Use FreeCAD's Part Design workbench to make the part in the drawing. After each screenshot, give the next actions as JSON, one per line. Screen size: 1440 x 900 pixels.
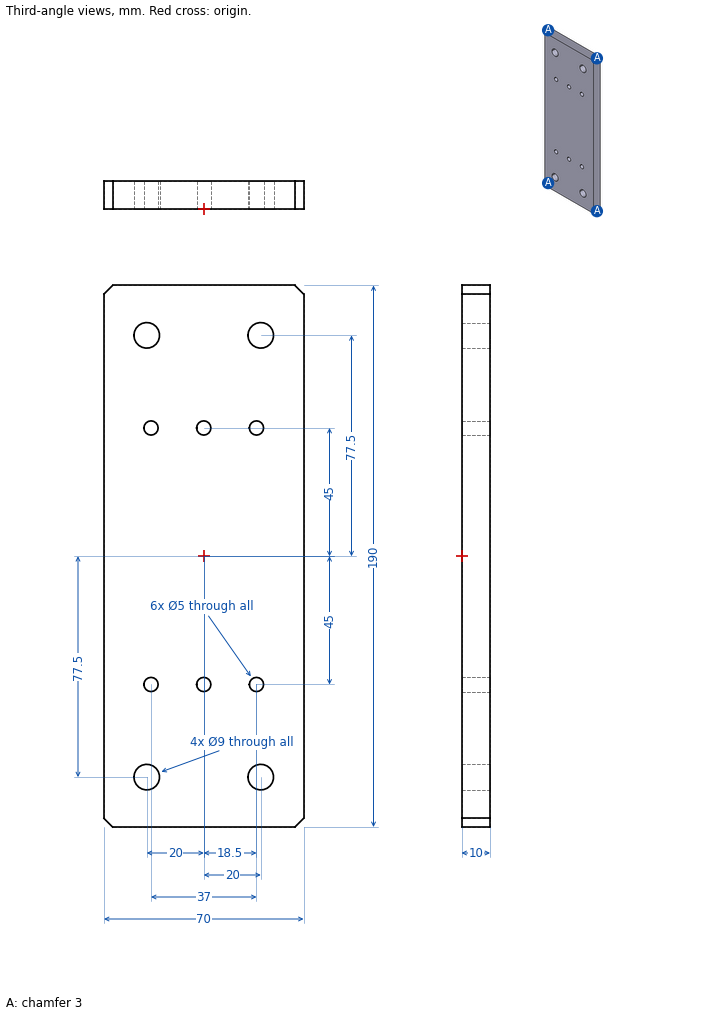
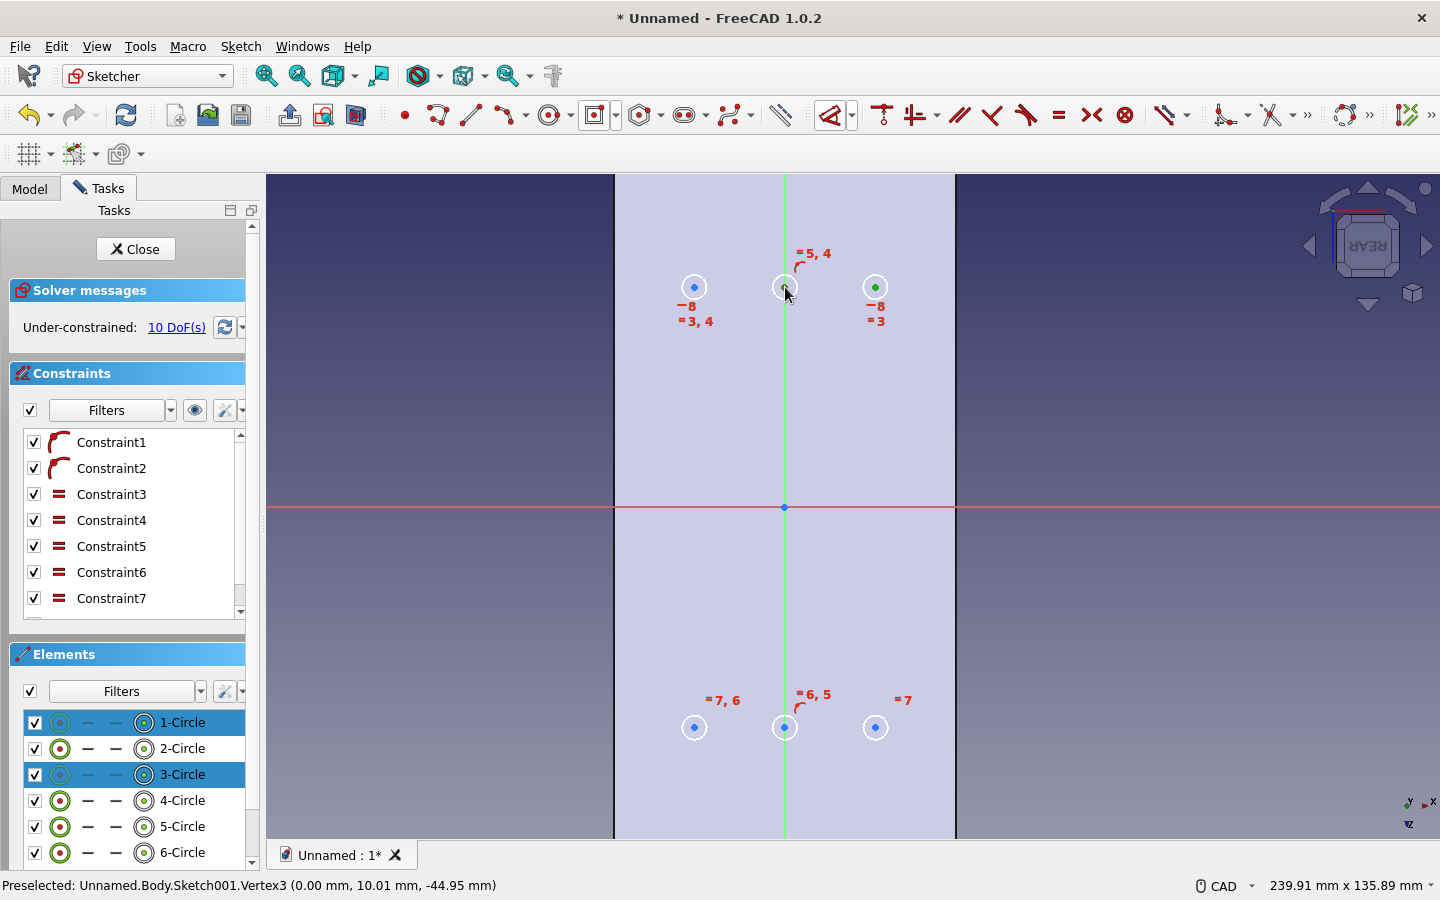
{"action": "left_click", "coordinate": [936, 116]}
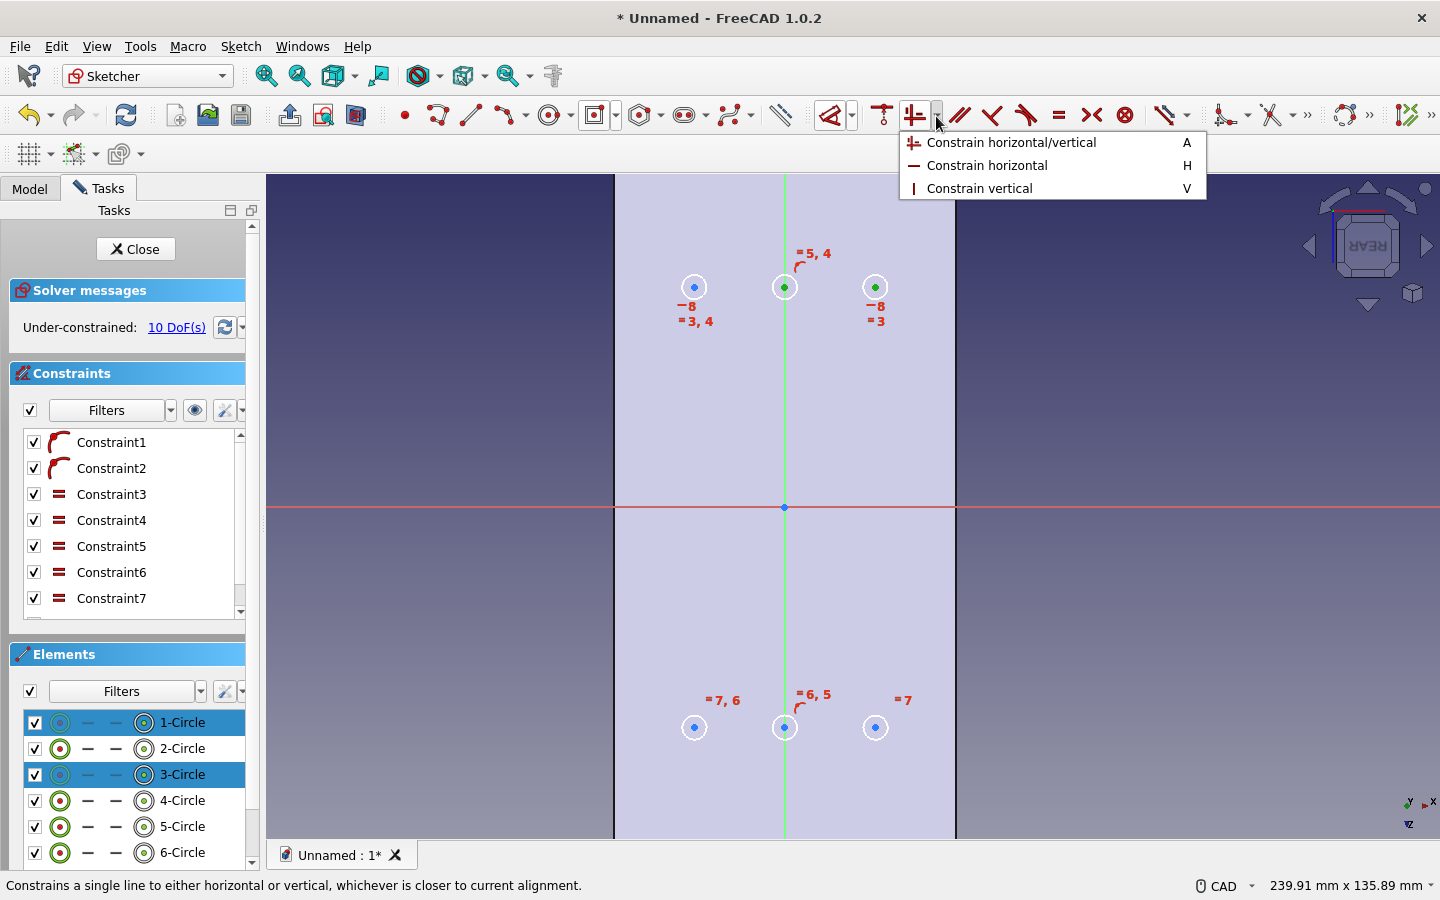
{"action": "left_click", "coordinate": [1053, 166]}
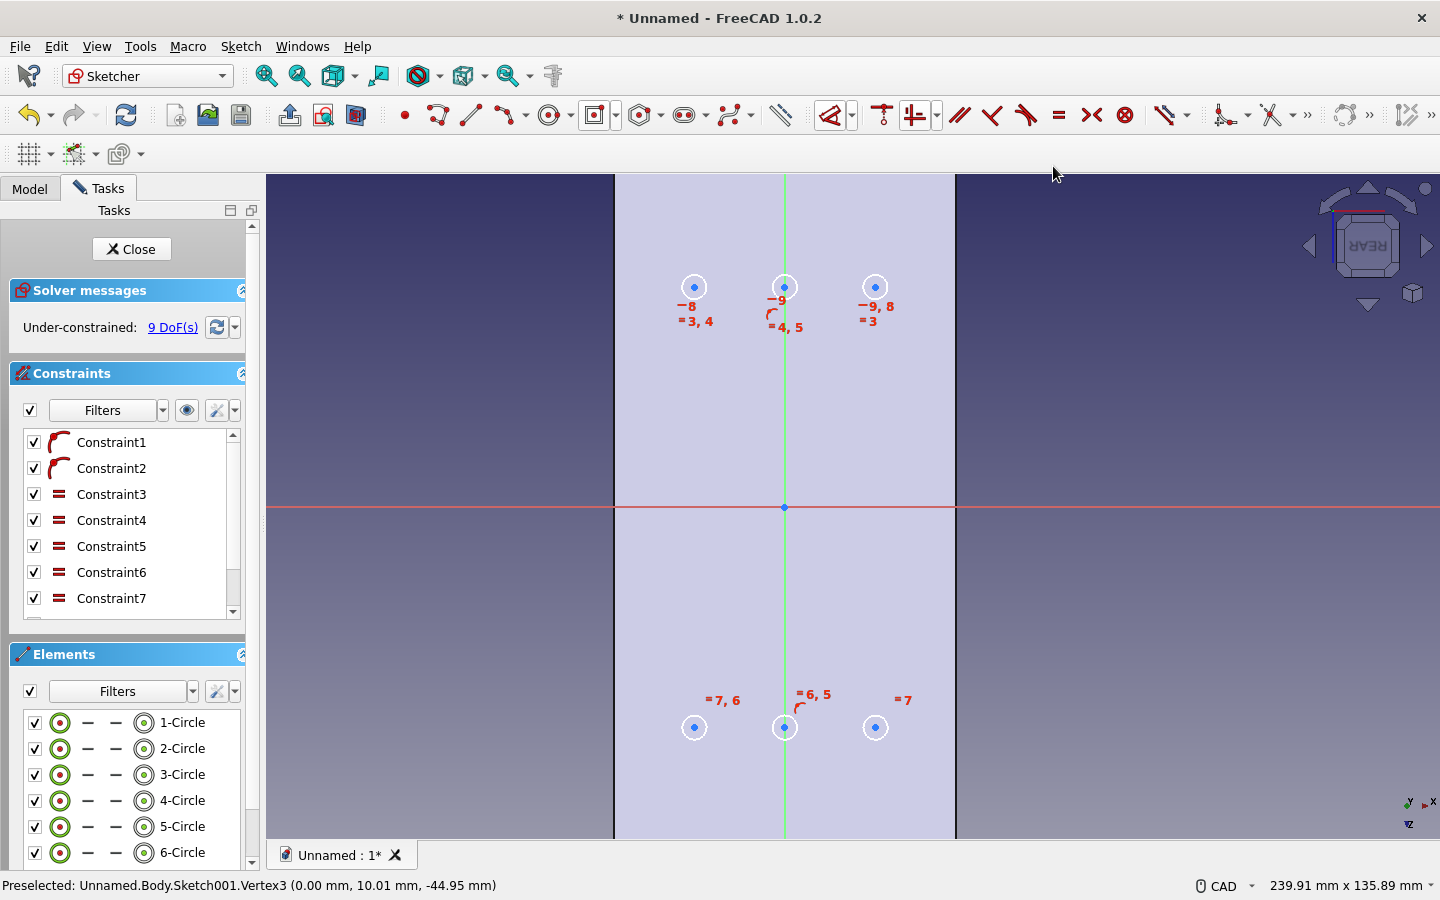
{"action": "left_click", "coordinate": [694, 287]}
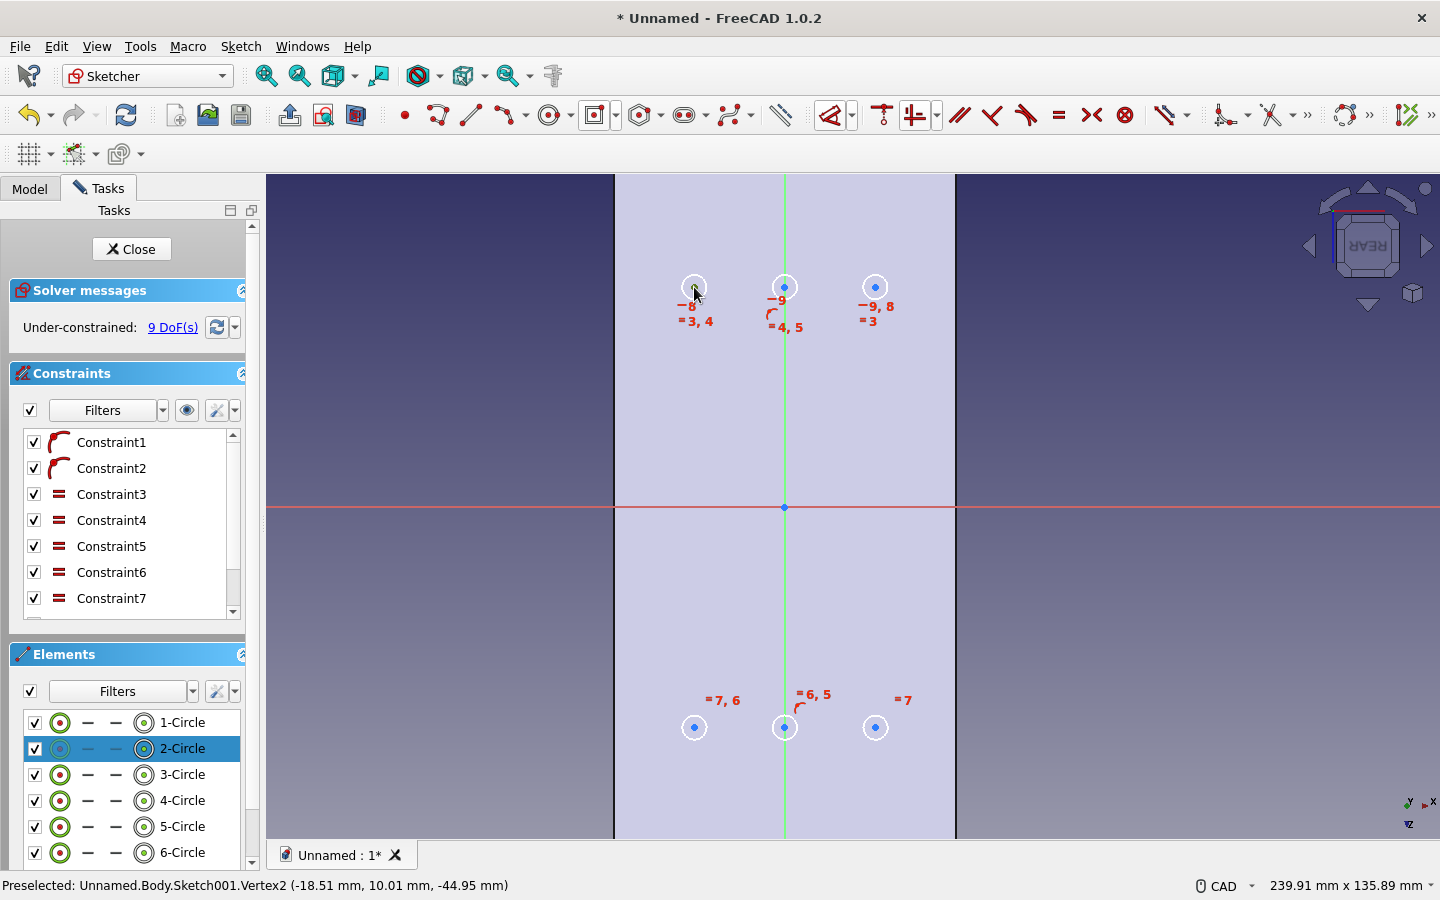
{"action": "left_click", "coordinate": [694, 728]}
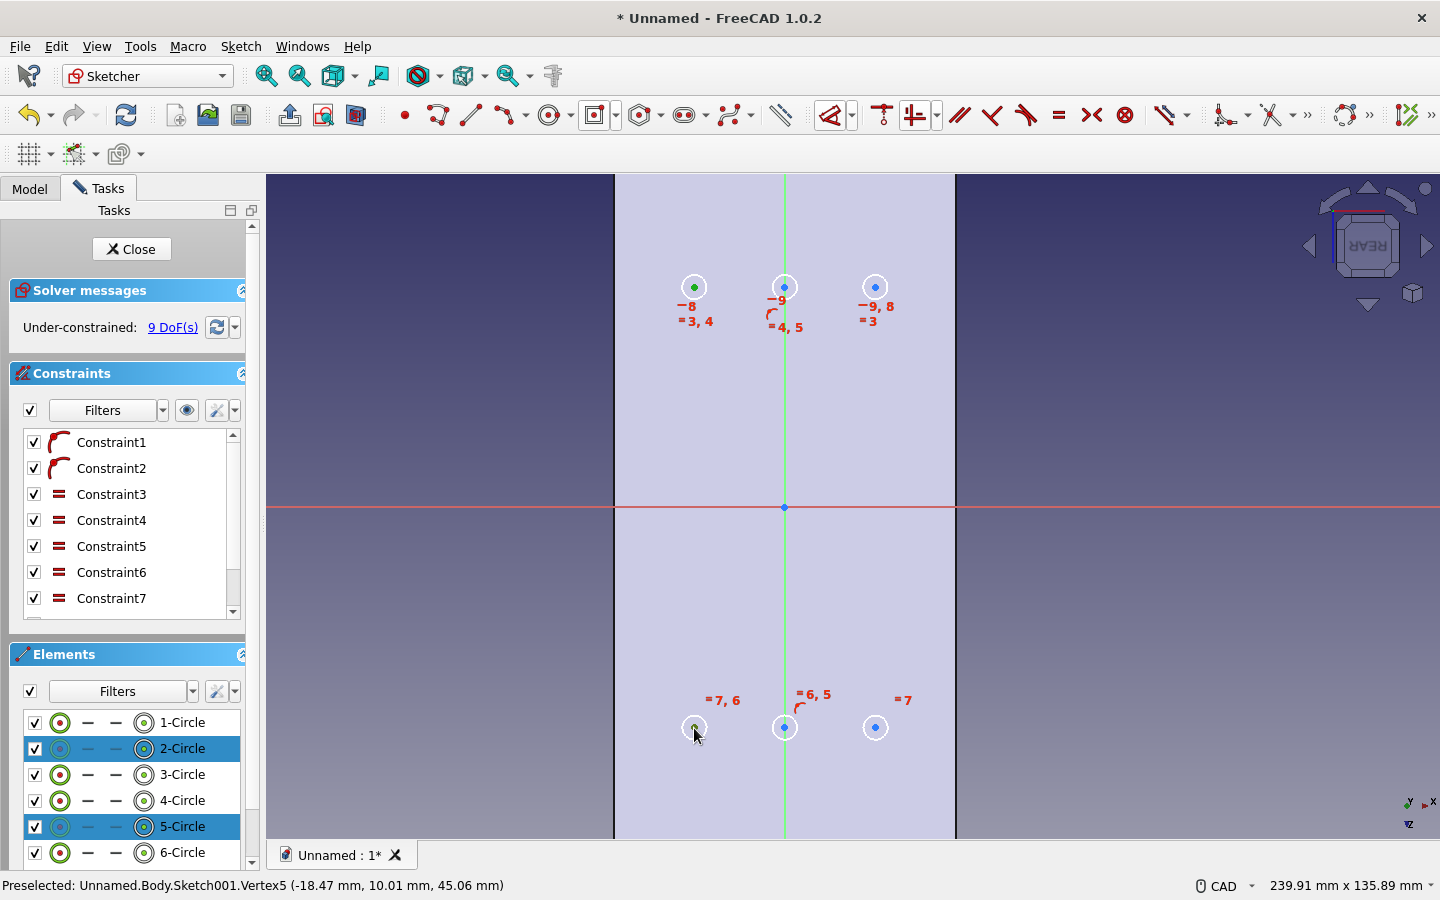
{"action": "key", "text": "v"}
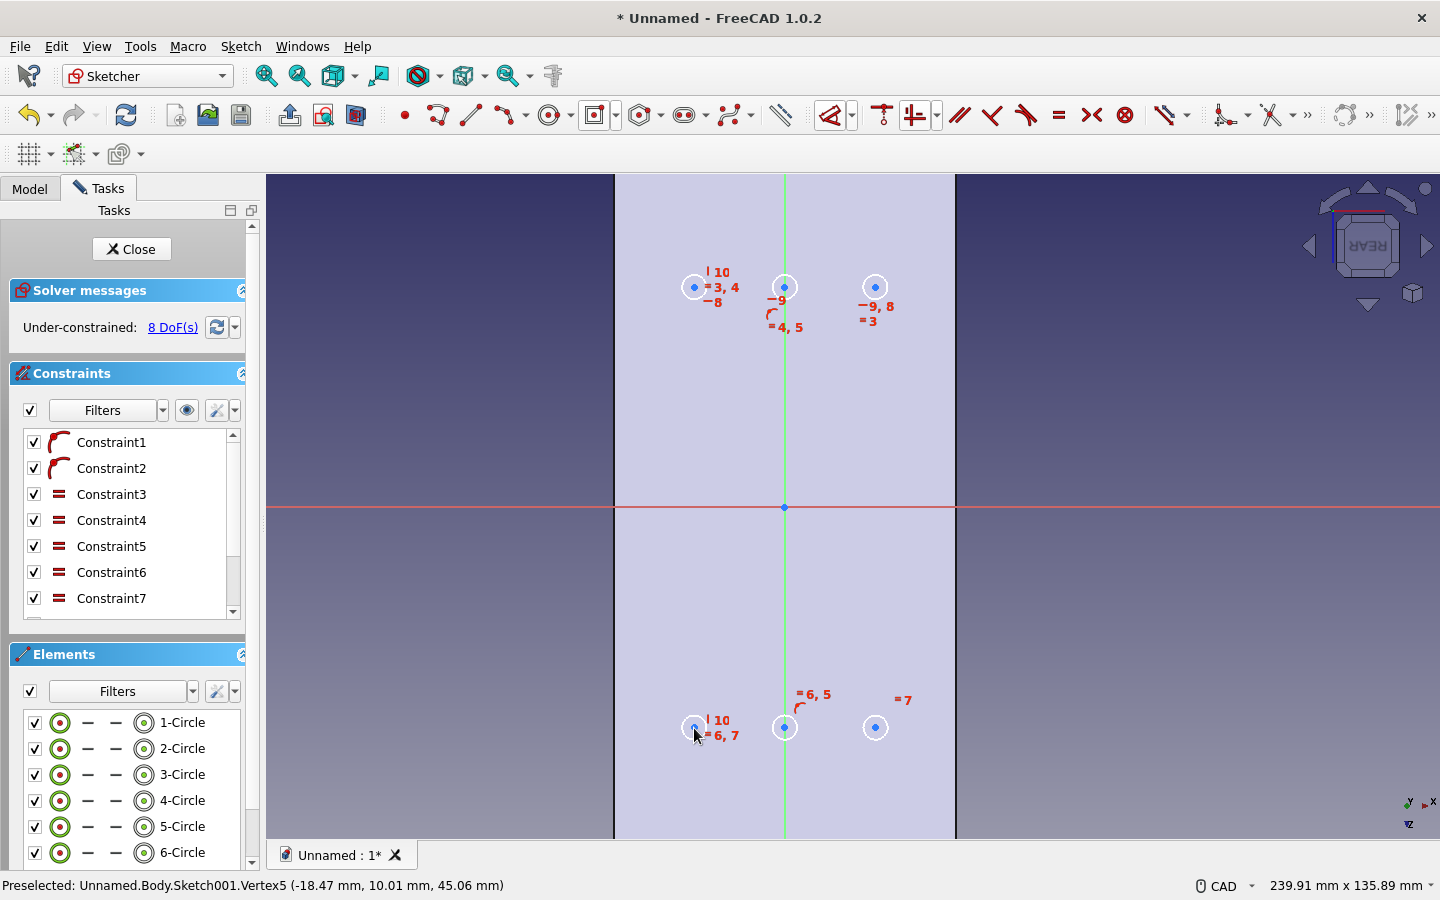
{"action": "left_click", "coordinate": [785, 728]}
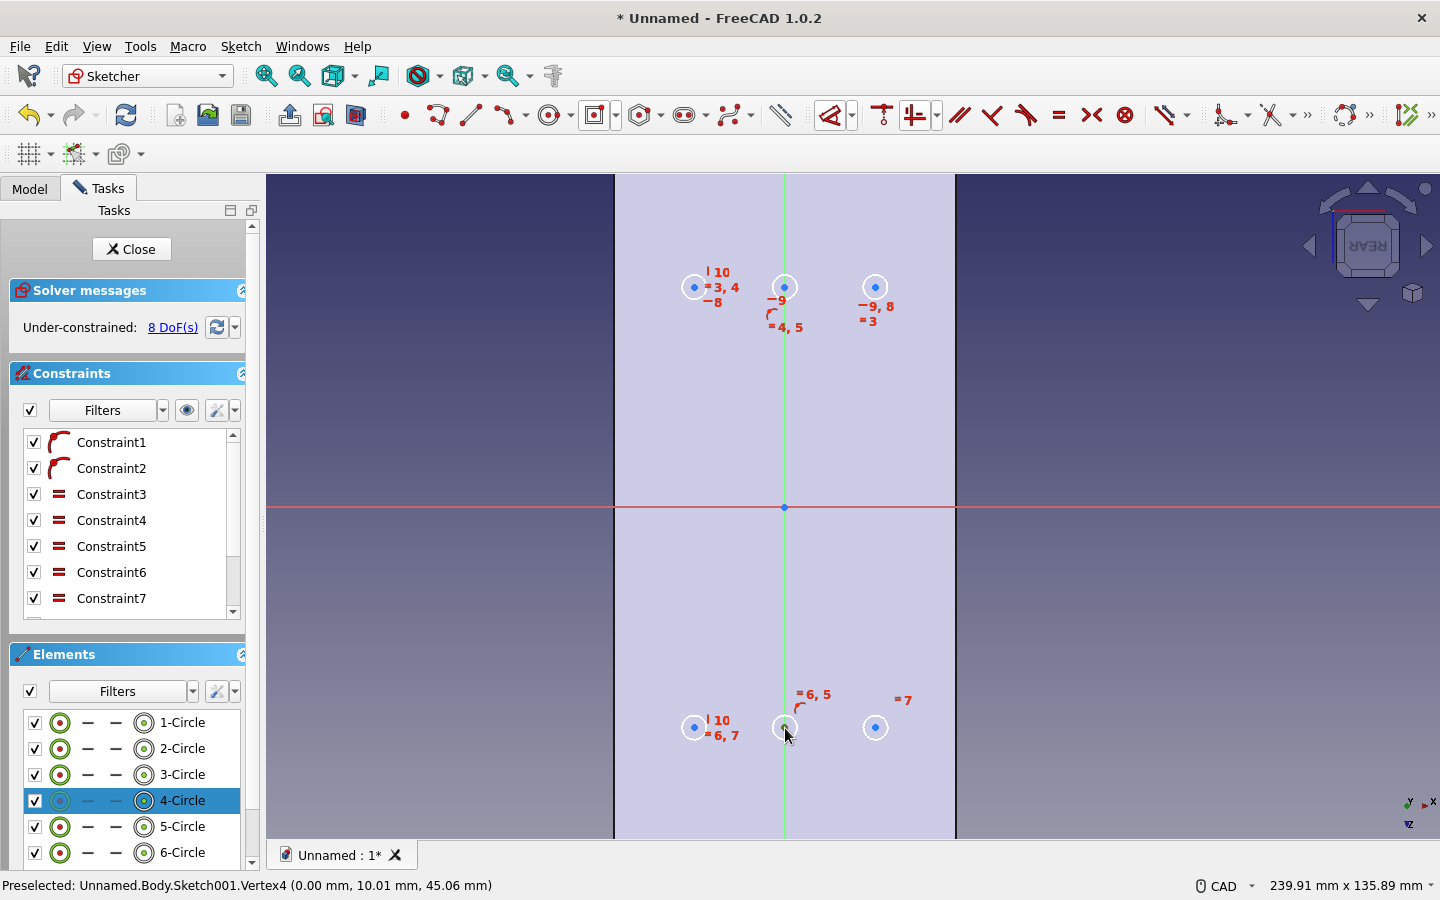
{"action": "left_click", "coordinate": [694, 728]}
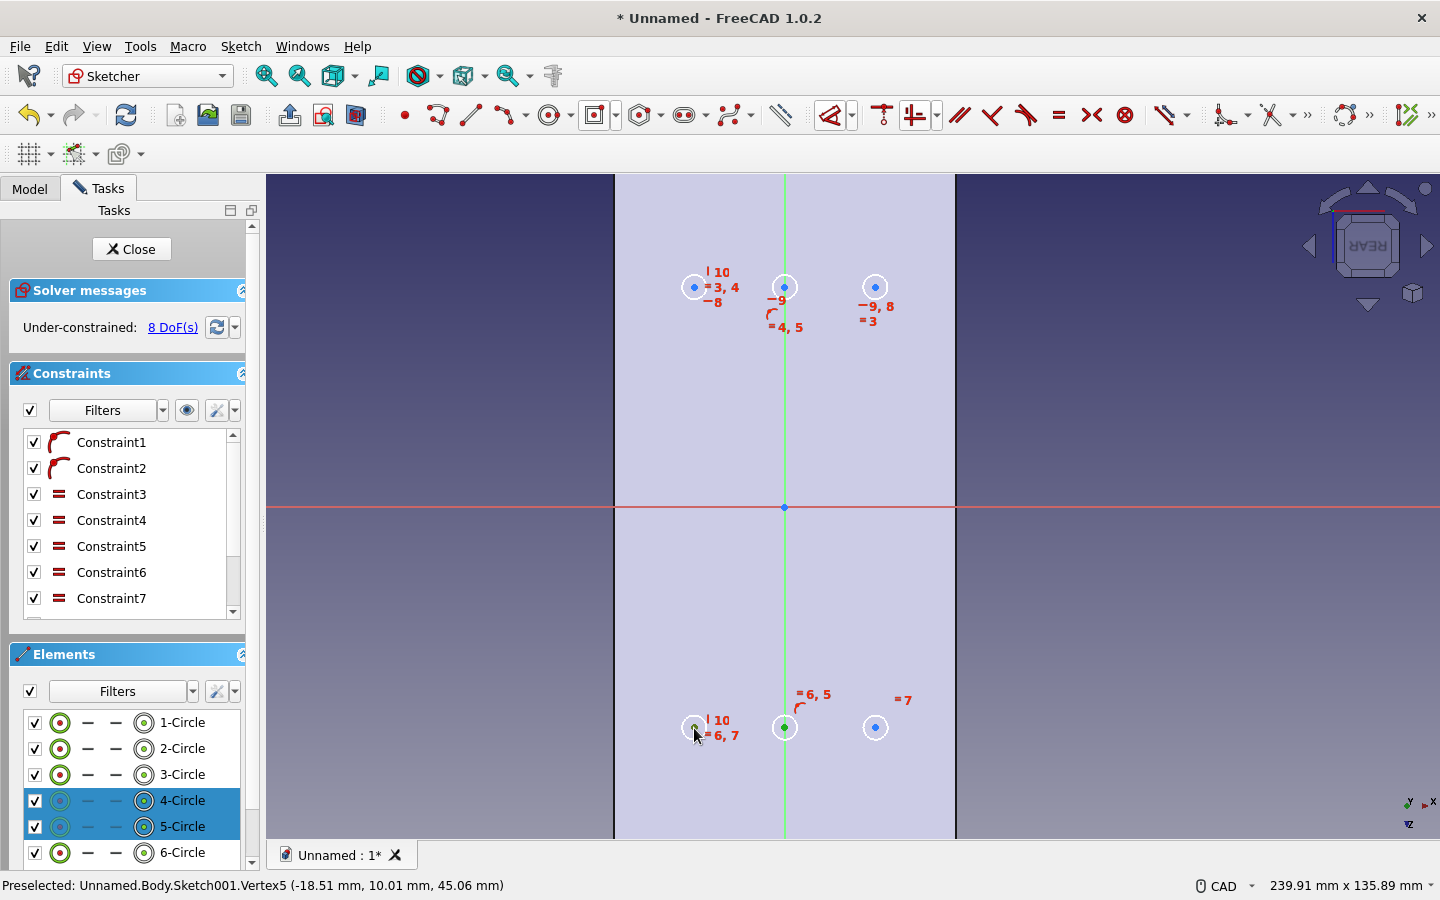
{"action": "left_click", "coordinate": [936, 116]}